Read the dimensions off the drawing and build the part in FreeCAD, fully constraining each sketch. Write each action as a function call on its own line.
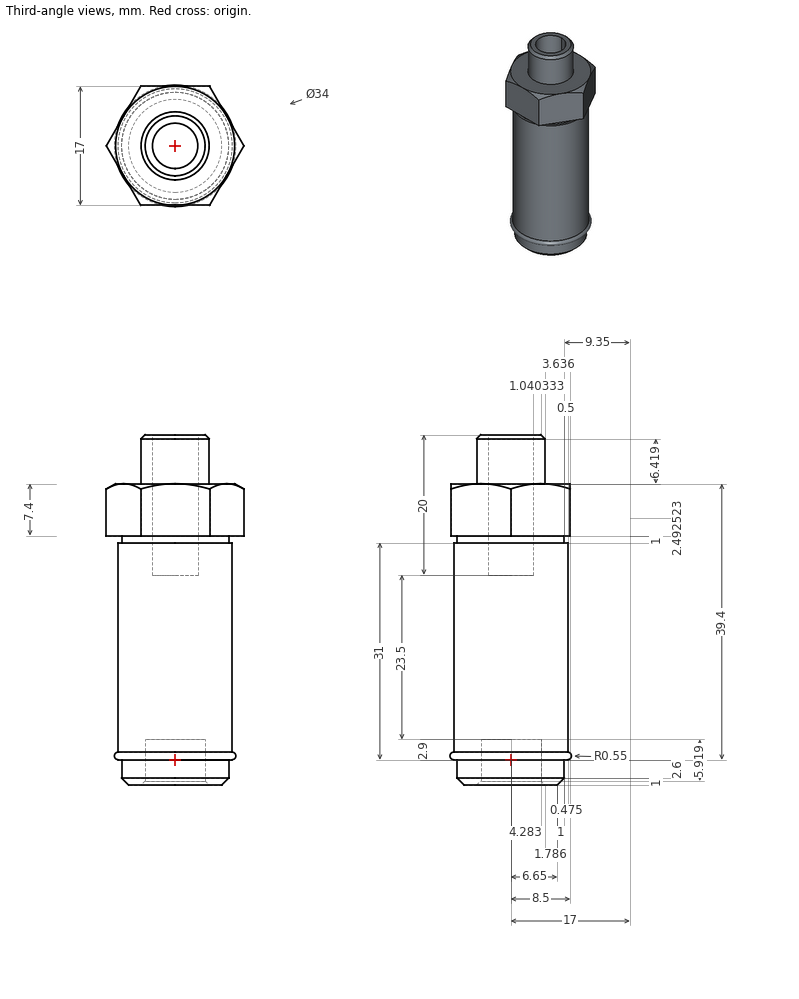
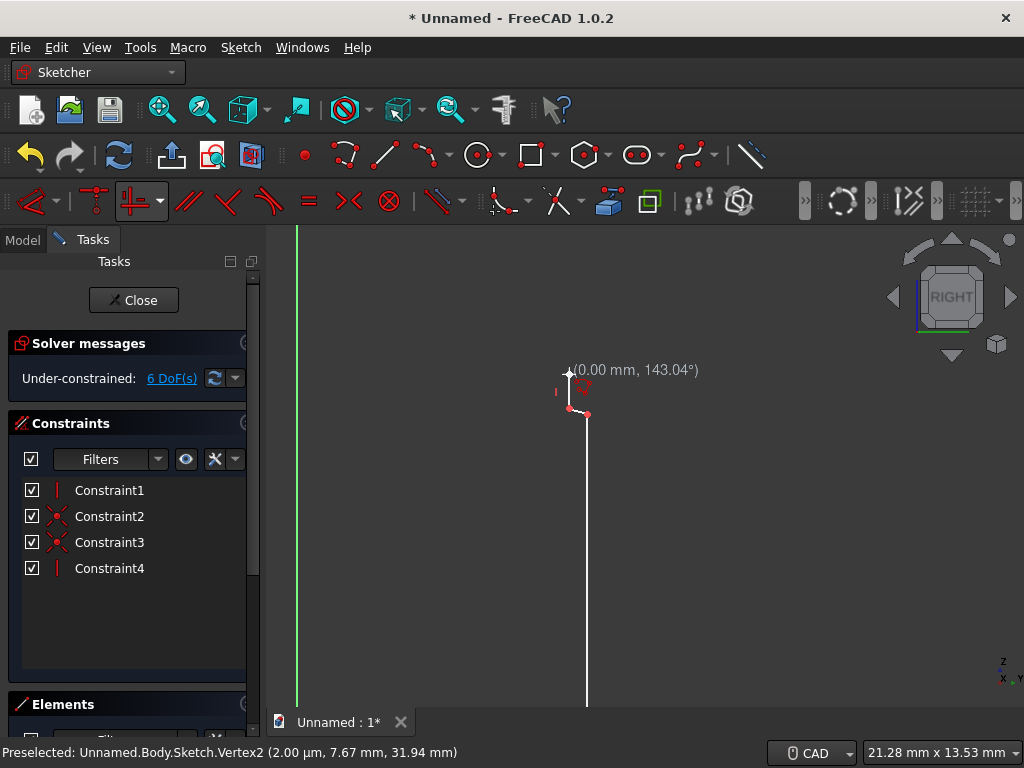
scroll(572, 409, down, 9)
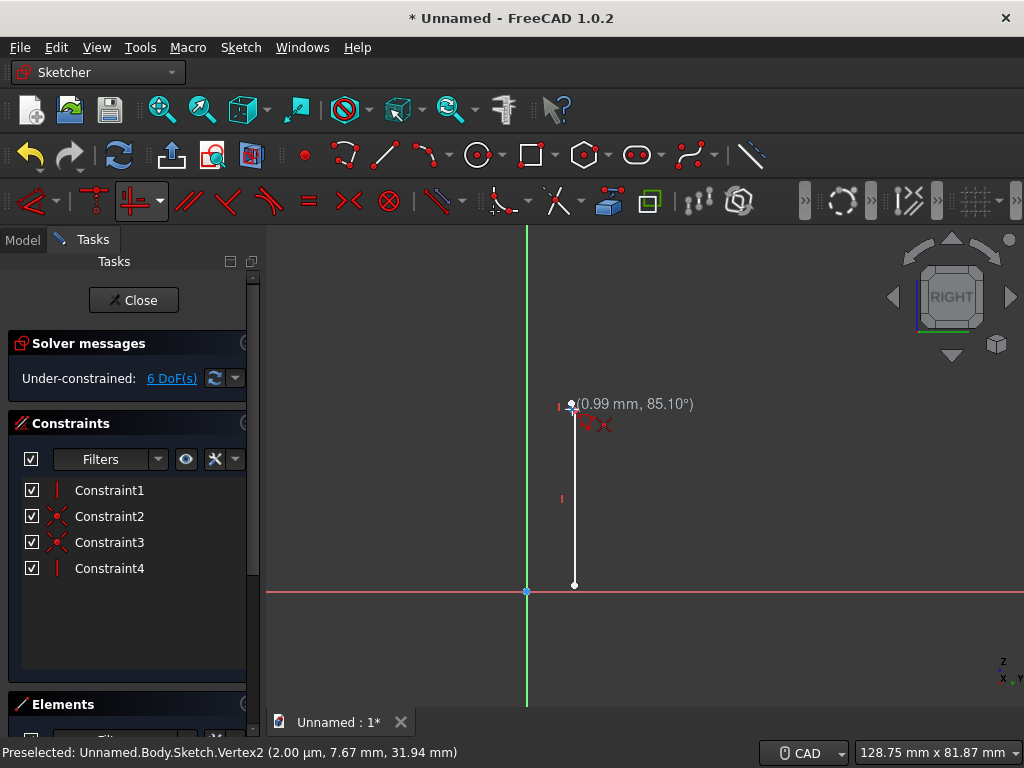
click(627, 404)
click(627, 389)
click(577, 360)
click(555, 360)
click(555, 322)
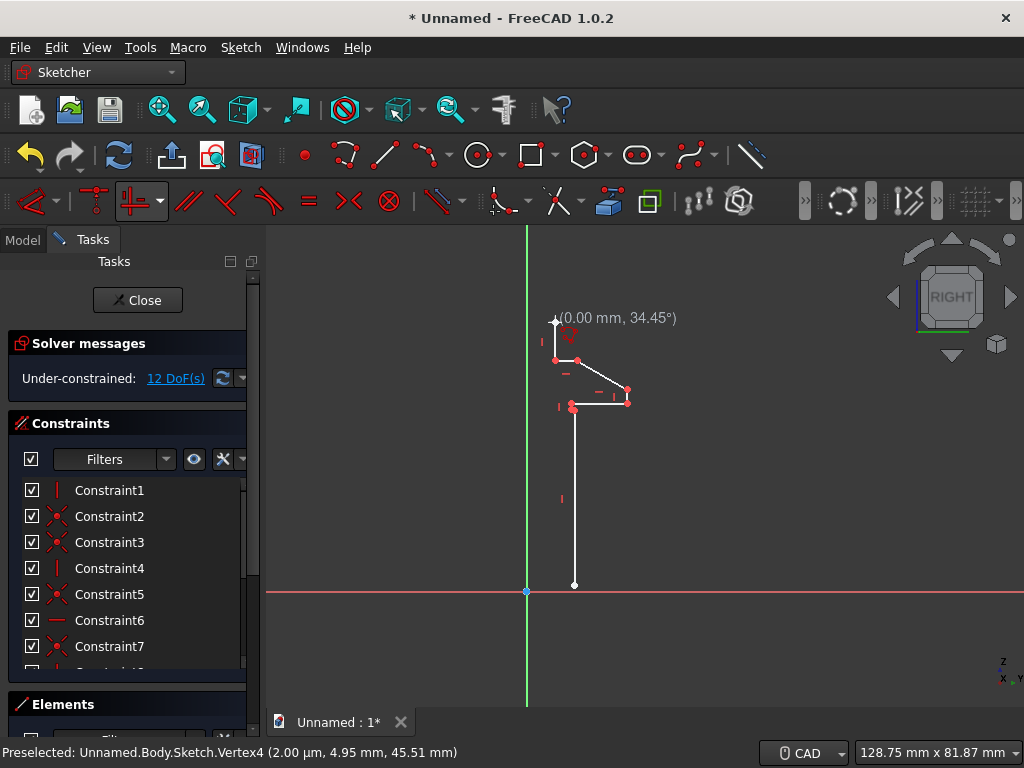
scroll(552, 319, up, 6)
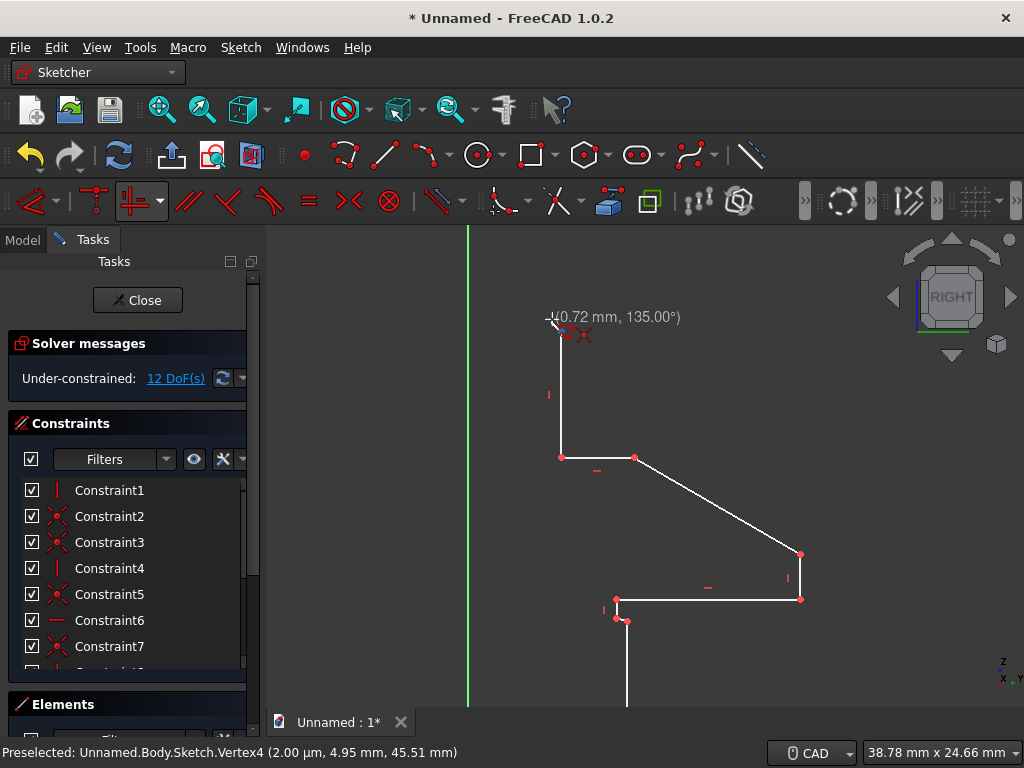
click(551, 318)
click(531, 318)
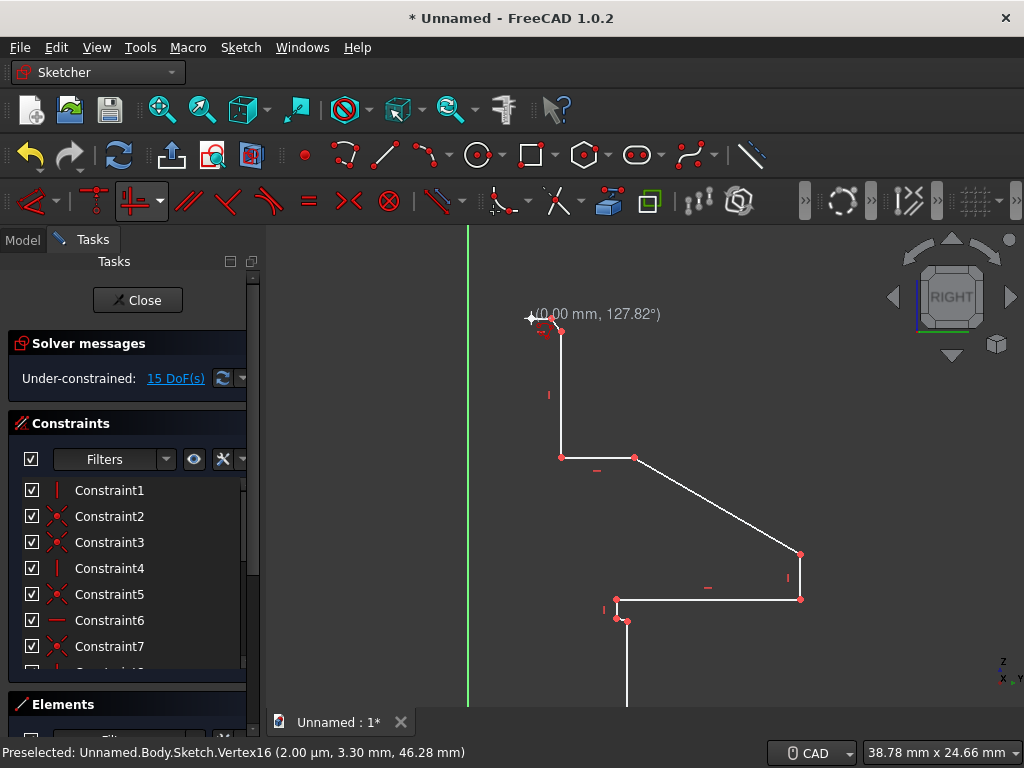
scroll(552, 319, down, 6)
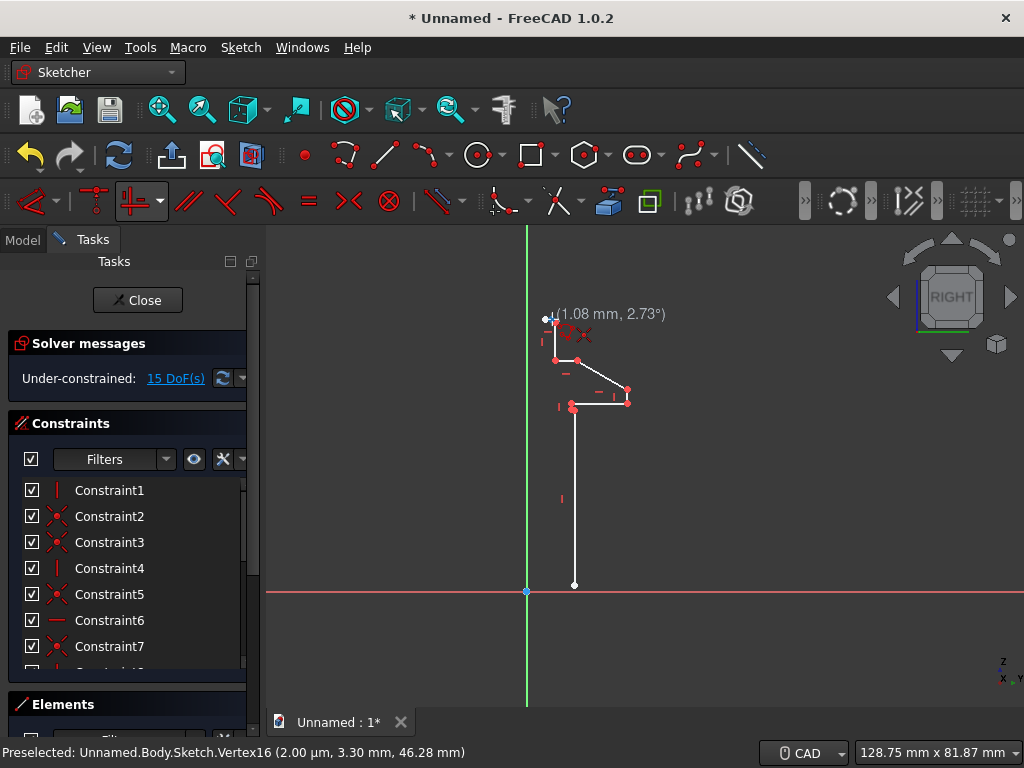
click(546, 436)
click(527, 436)
click(536, 575)
click(552, 575)
click(552, 610)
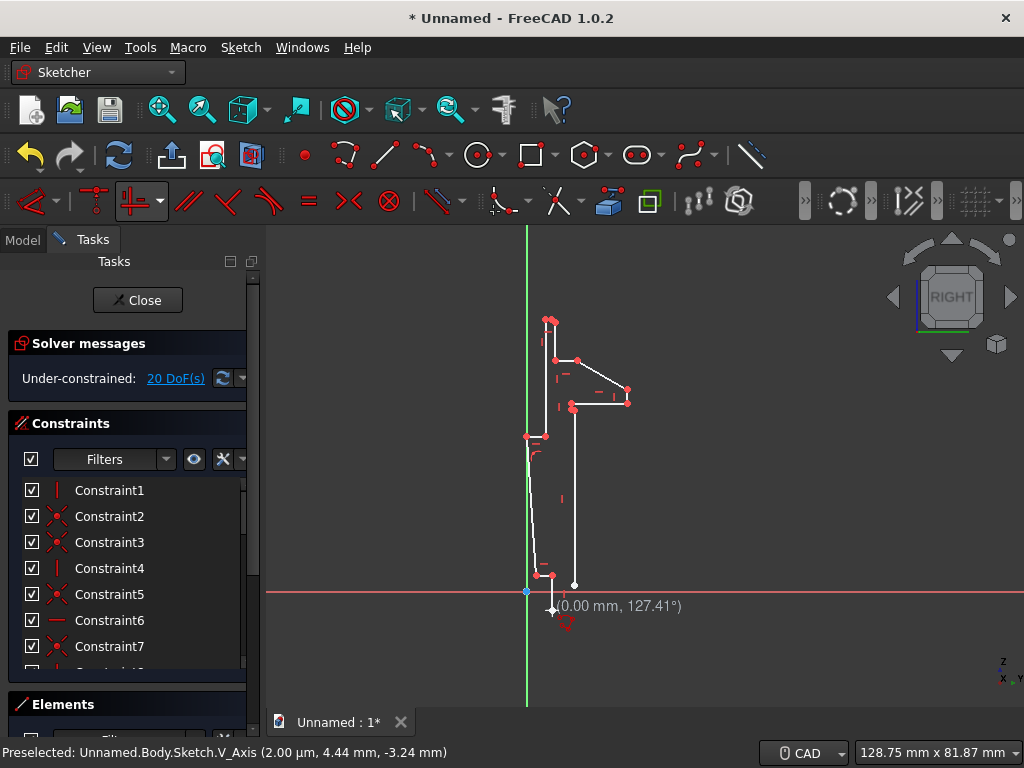
scroll(555, 613, up, 6)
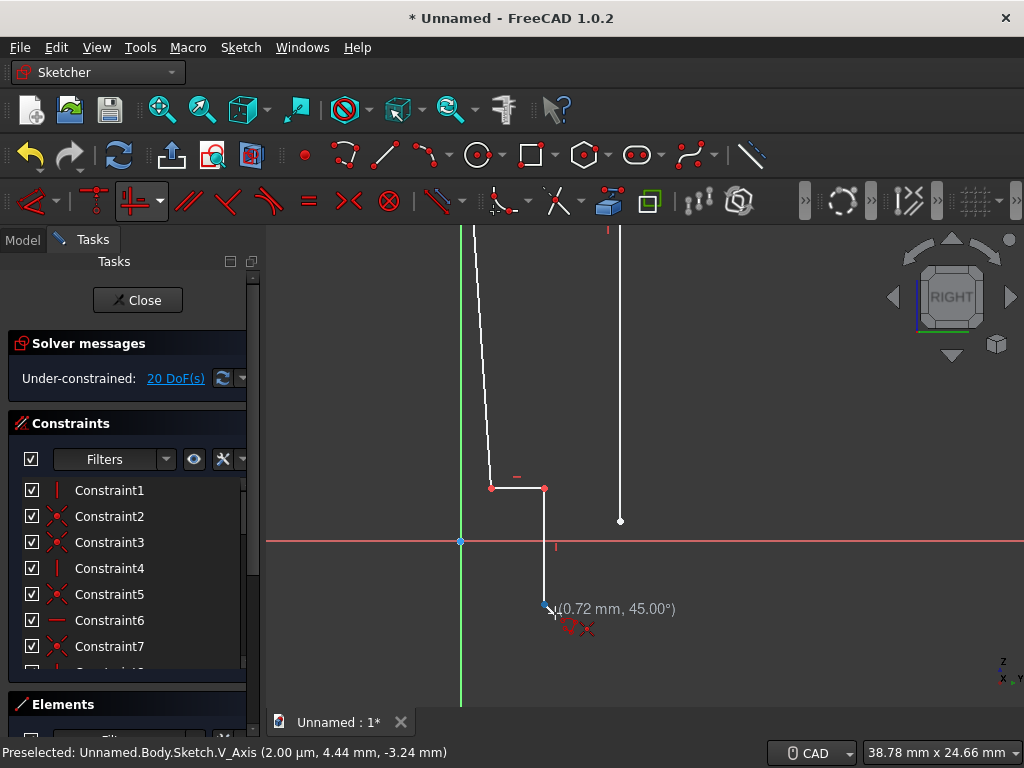
click(556, 611)
click(591, 611)
click(610, 592)
click(610, 541)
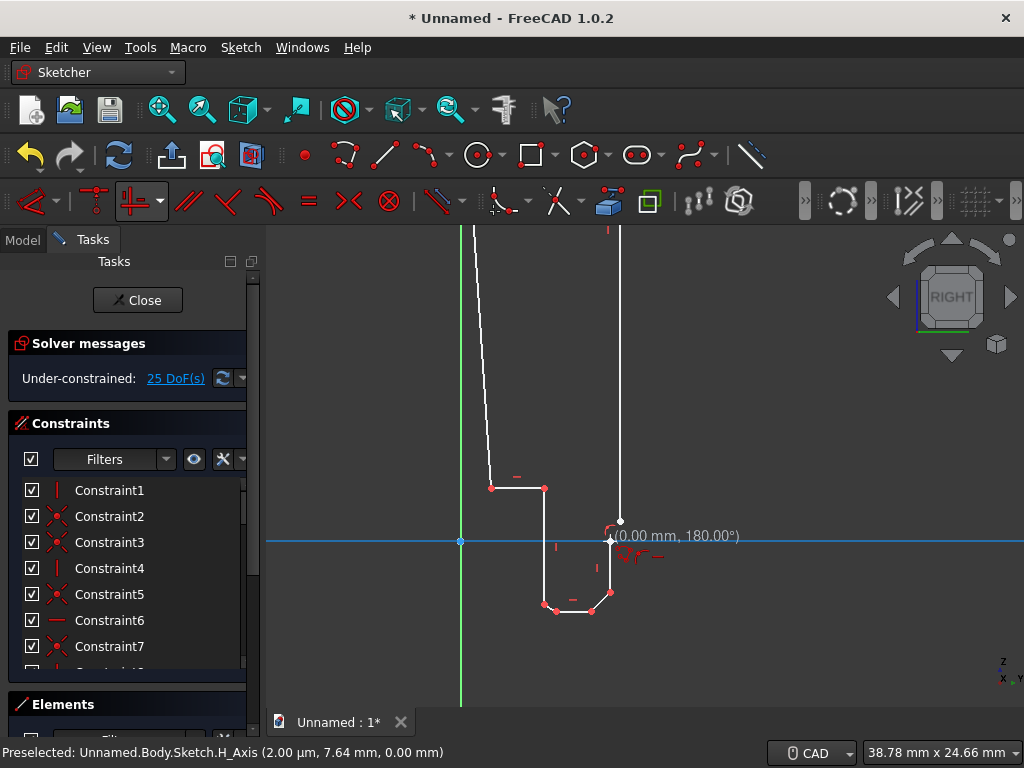
scroll(619, 541, up, 3)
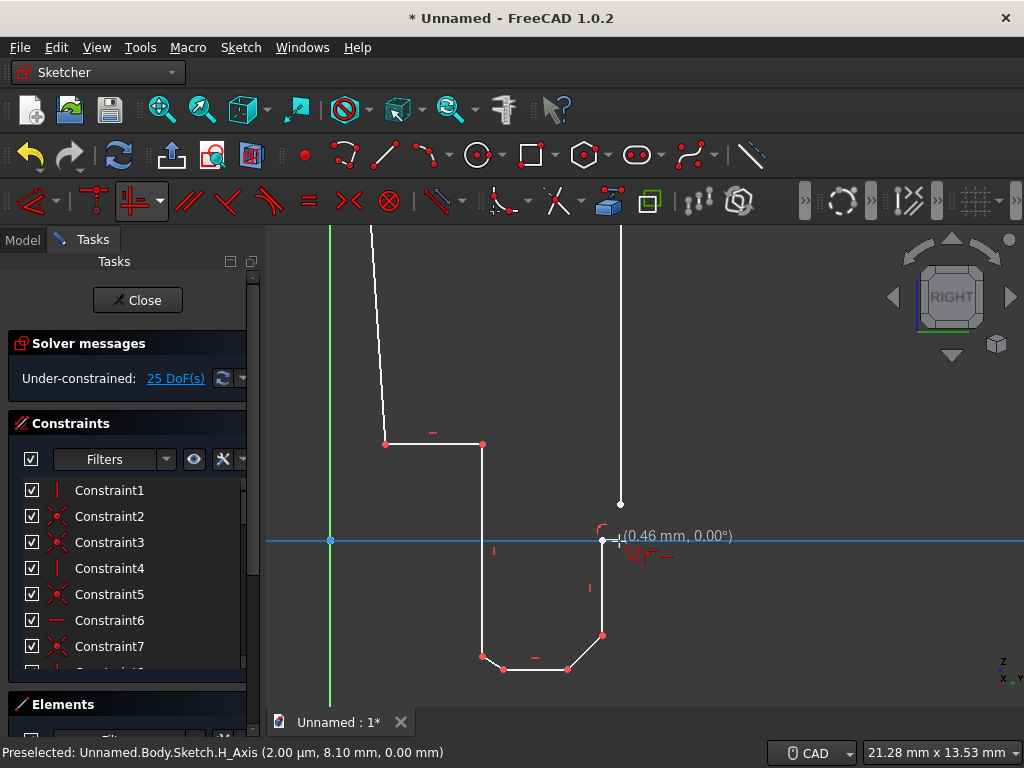
click(619, 532)
right_click(619, 532)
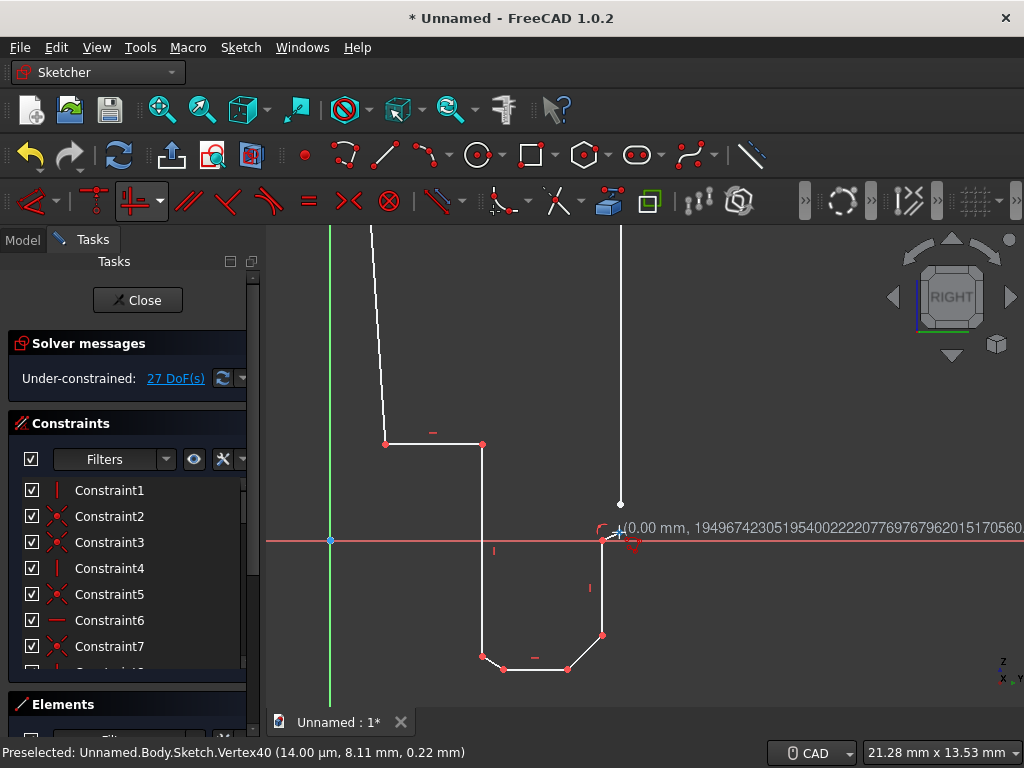
key(g)
key(3)
key(a)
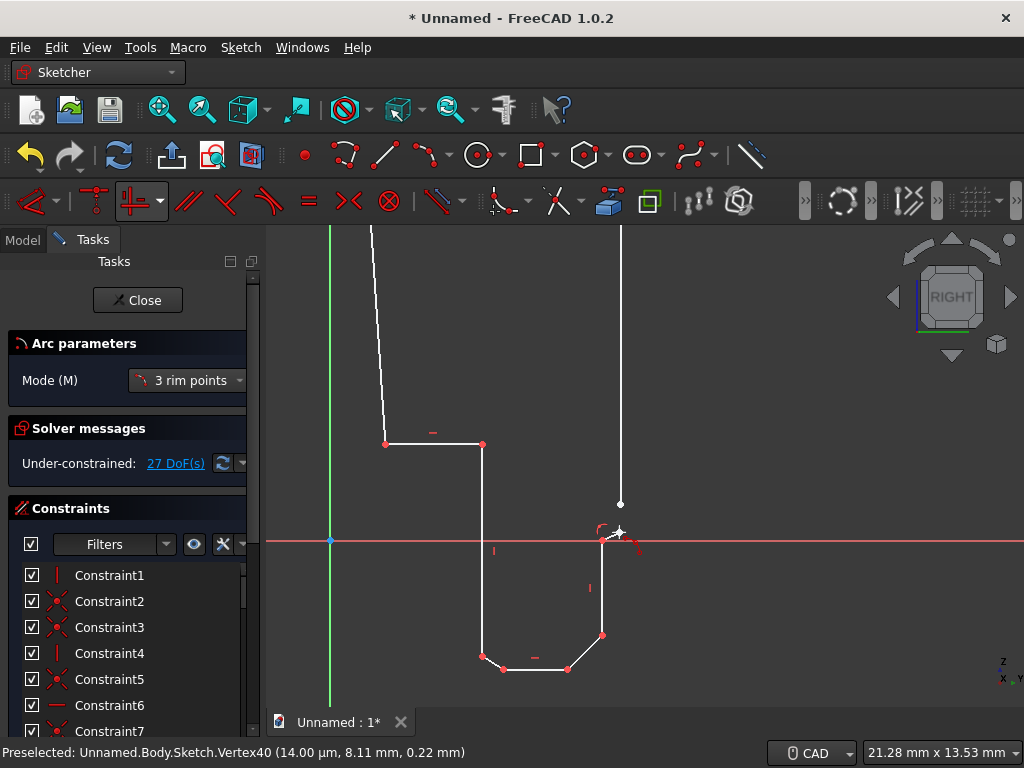
scroll(619, 541, up, 4)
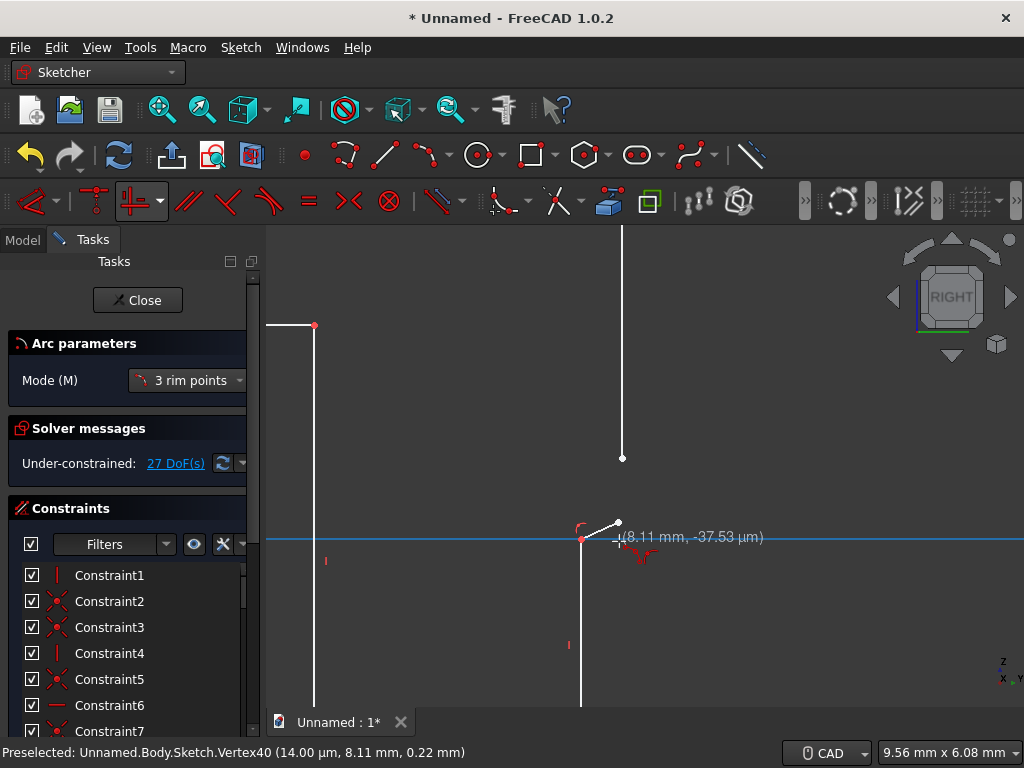
click(618, 522)